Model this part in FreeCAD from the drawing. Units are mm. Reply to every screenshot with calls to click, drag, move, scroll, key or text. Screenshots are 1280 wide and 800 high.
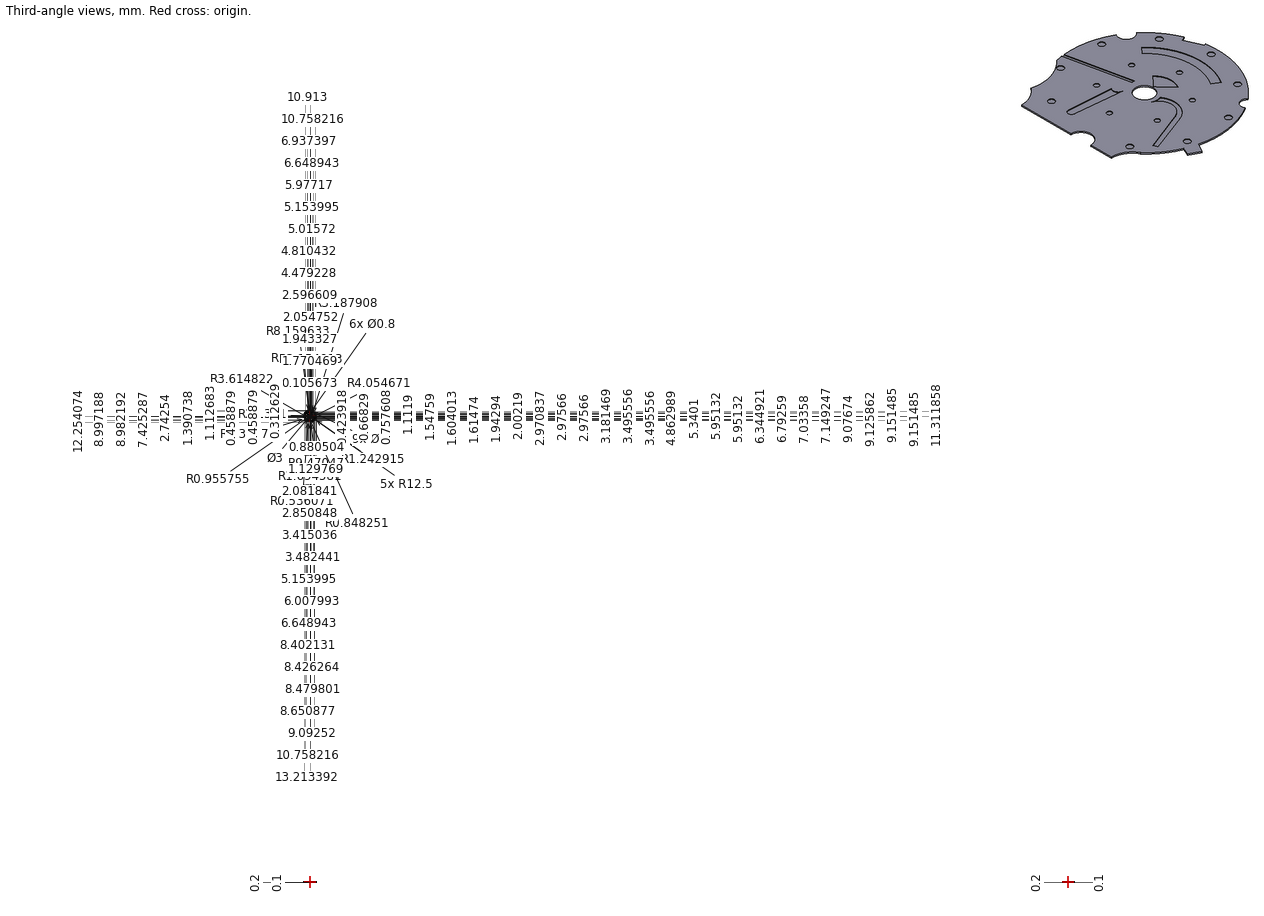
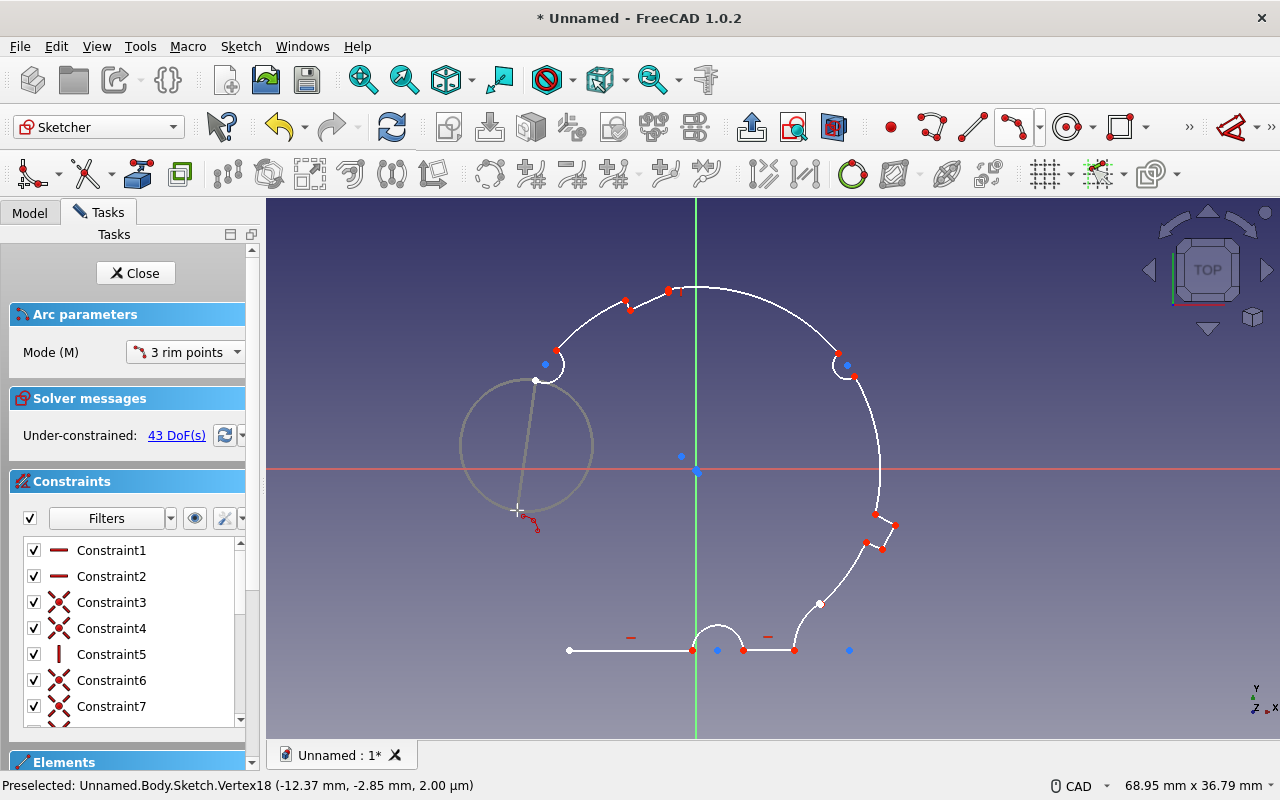
scroll(514, 443, up, 2)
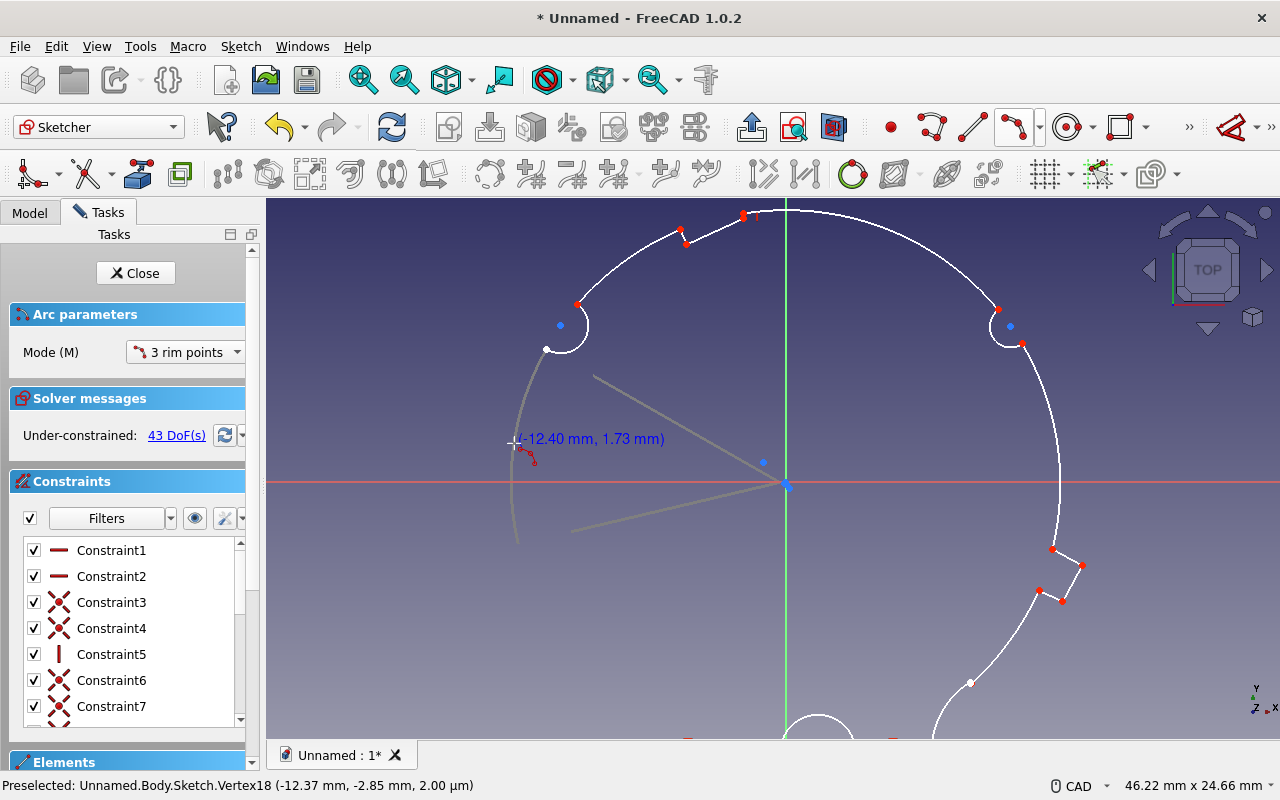
click(515, 443)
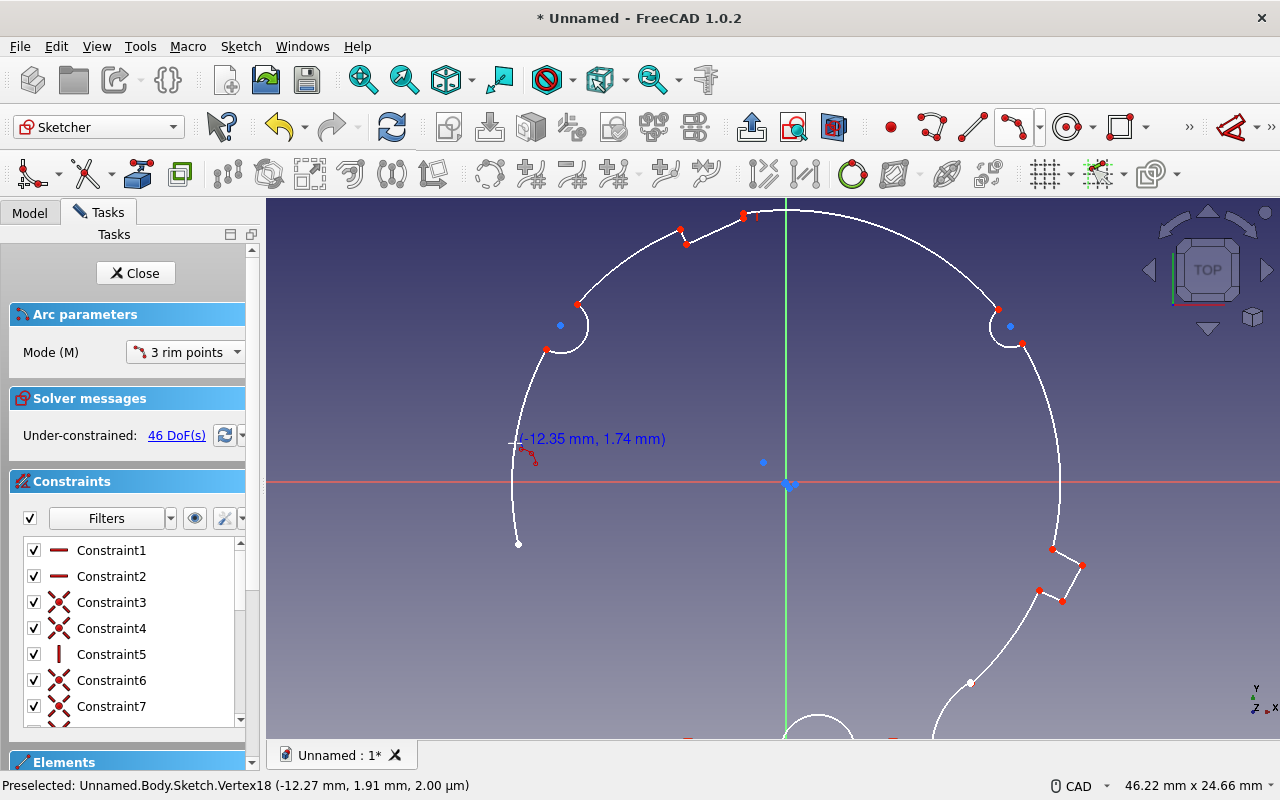
click(518, 544)
click(560, 679)
click(558, 605)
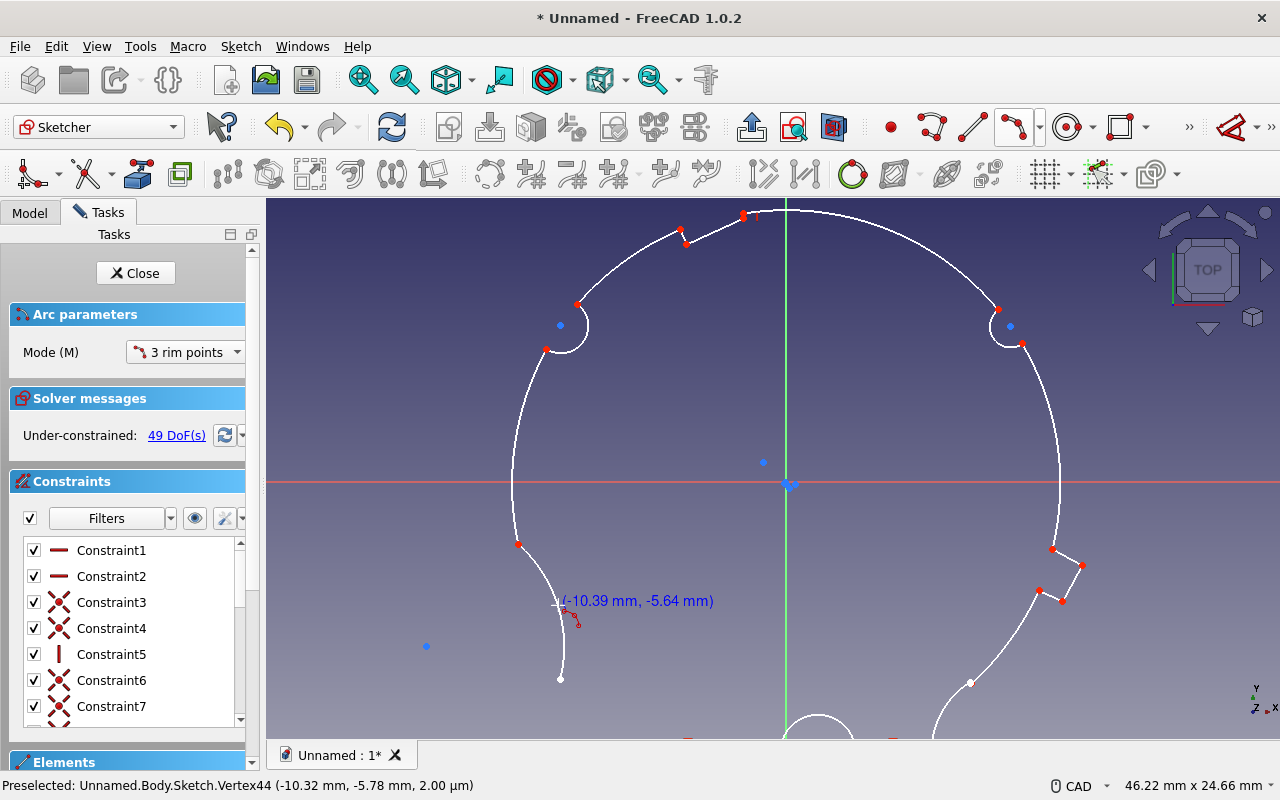
click(560, 680)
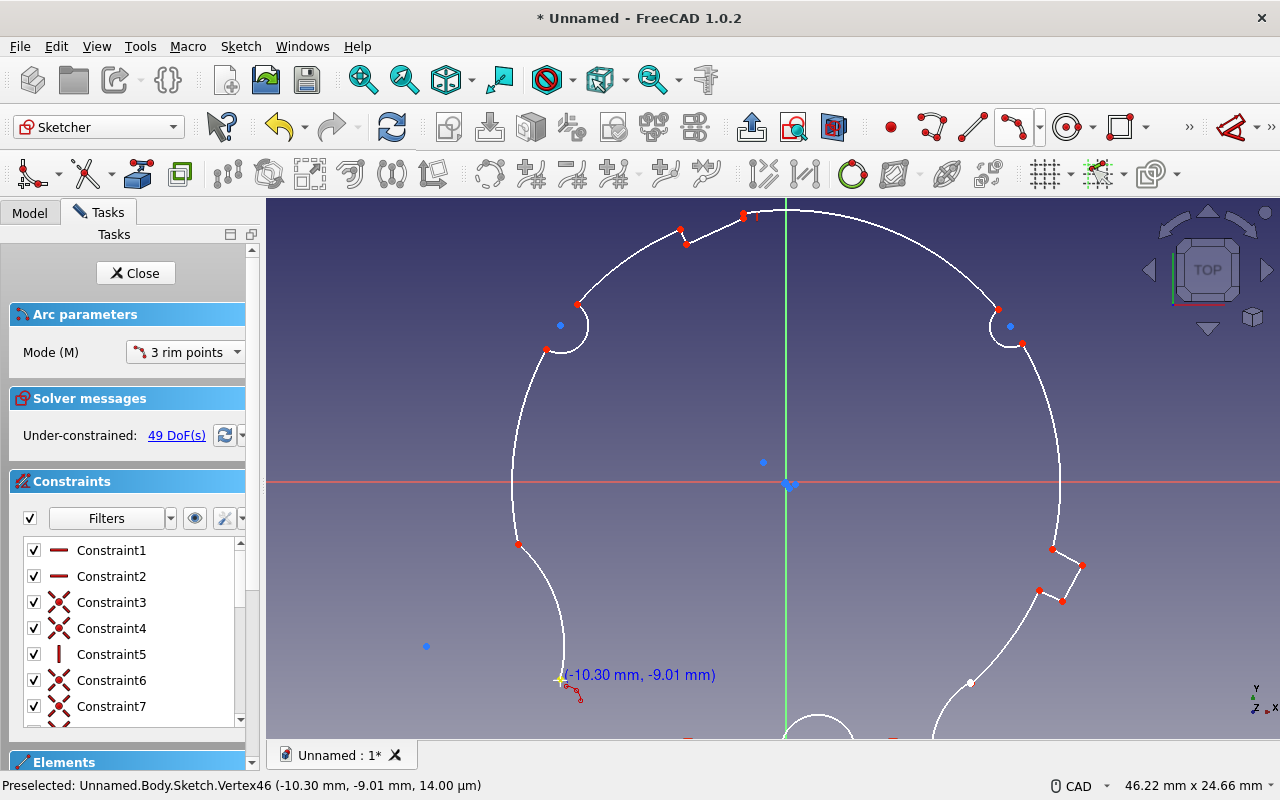
scroll(513, 443, down, 2)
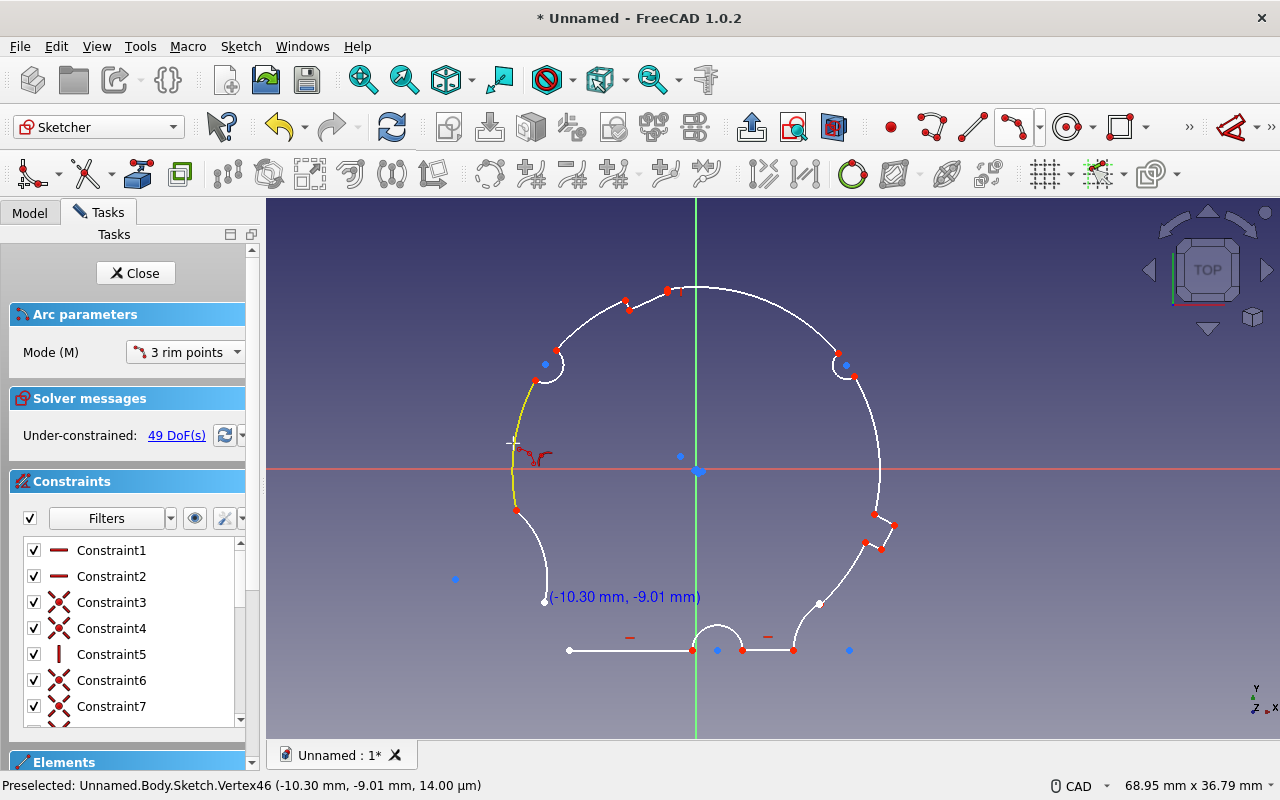
click(569, 651)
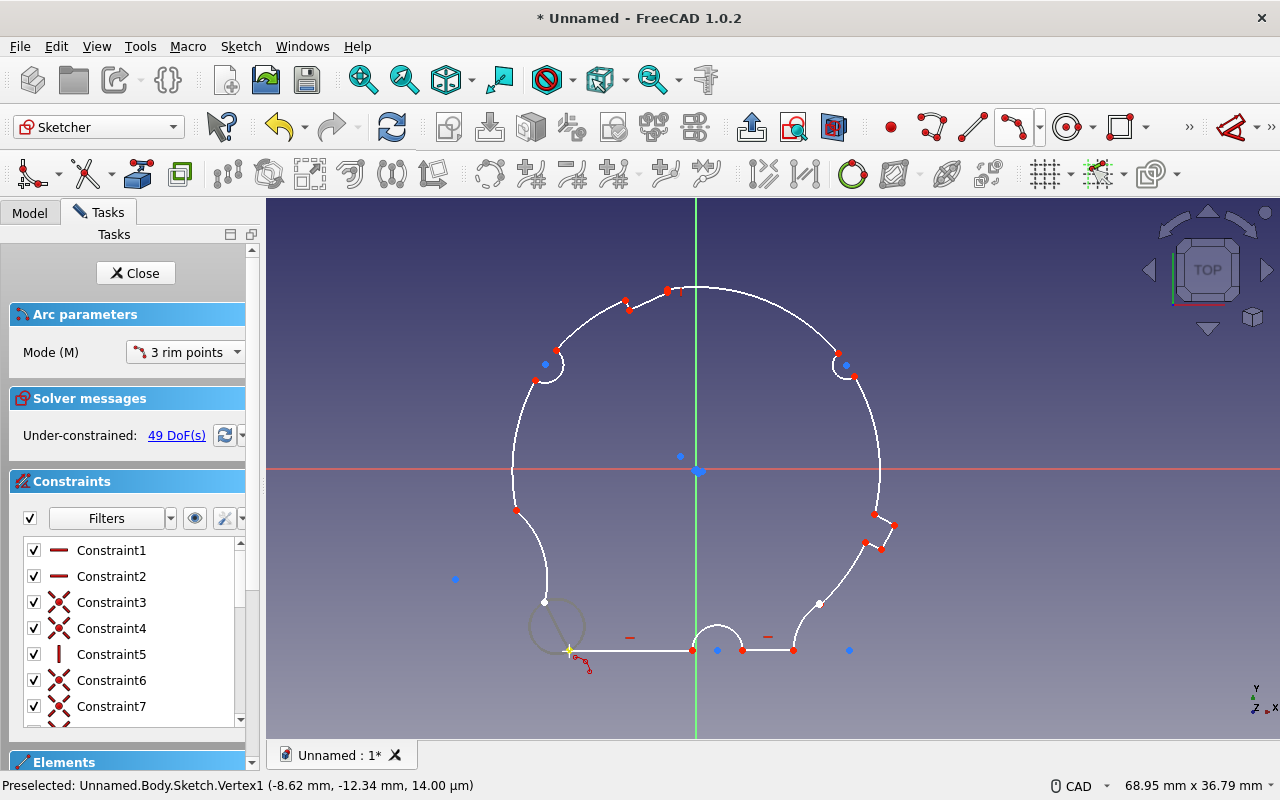
scroll(562, 623, up, 5)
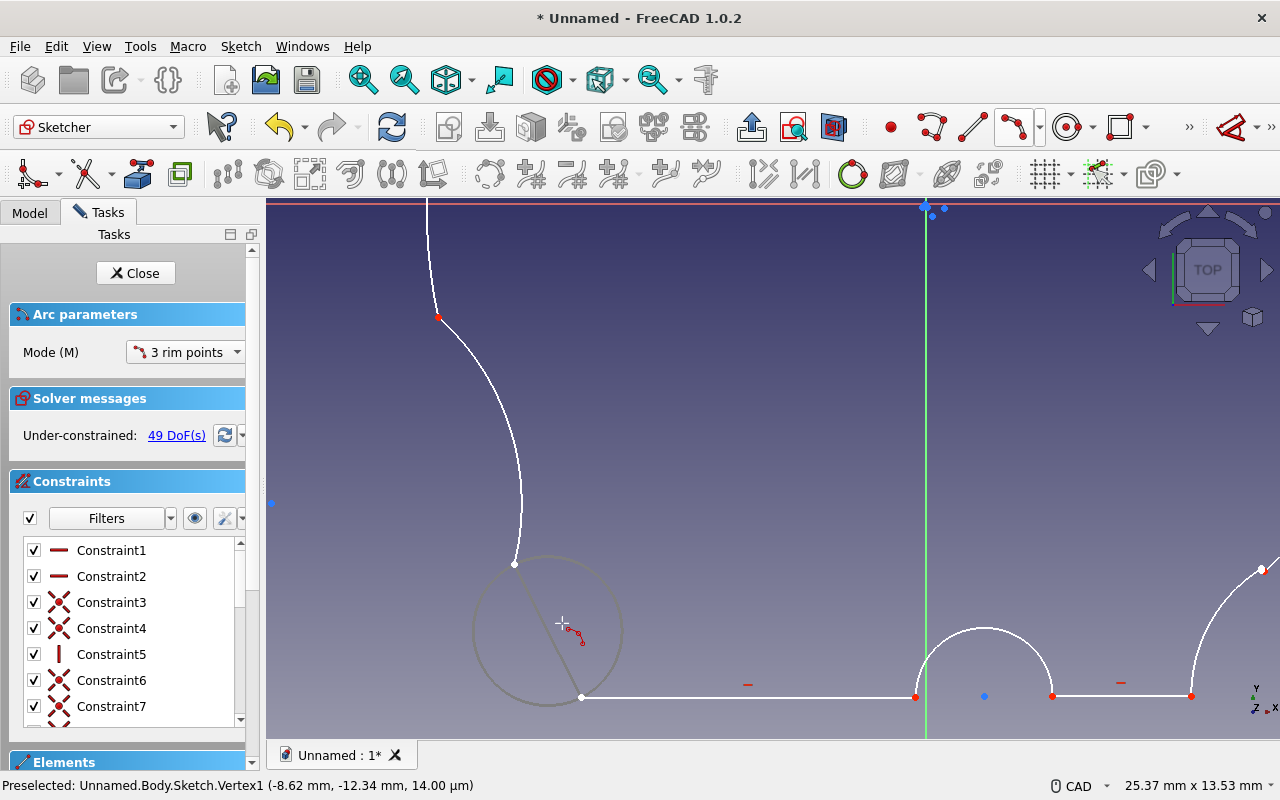
click(562, 621)
key(Escape)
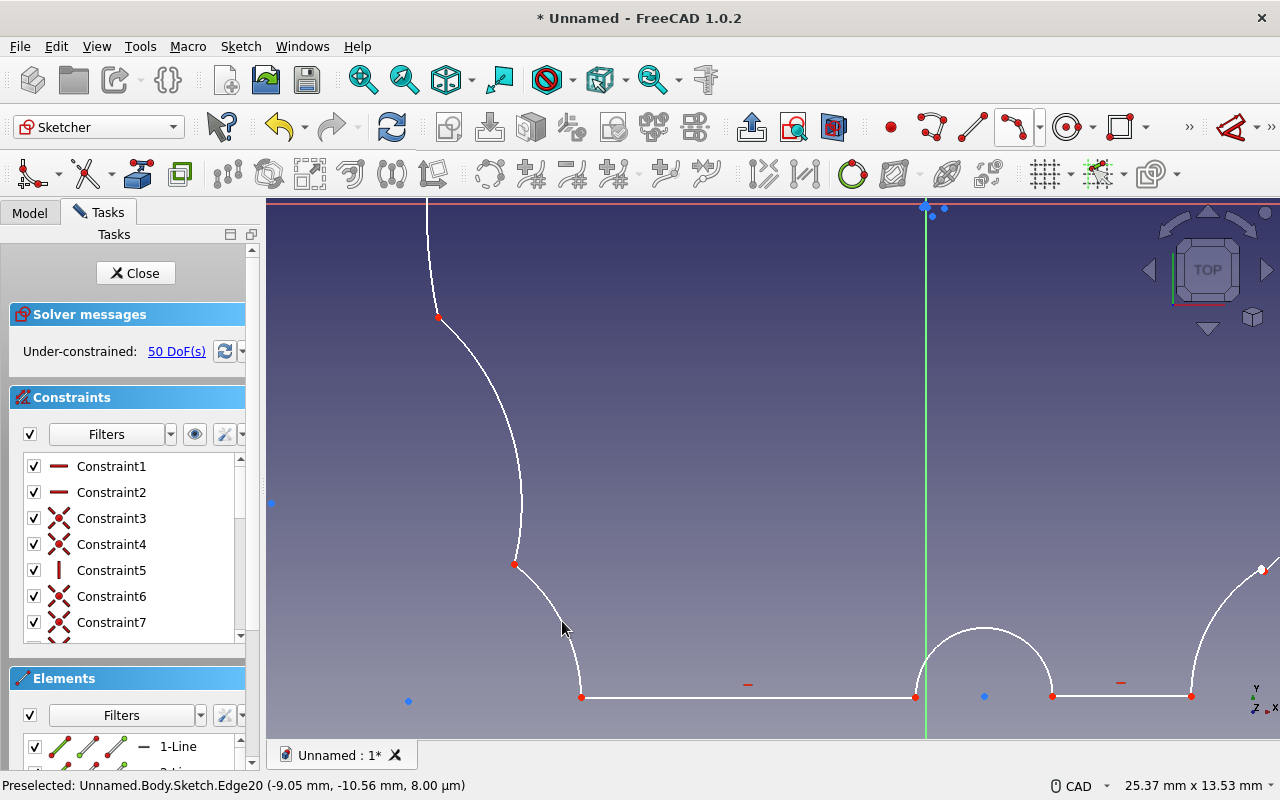
scroll(562, 623, down, 5)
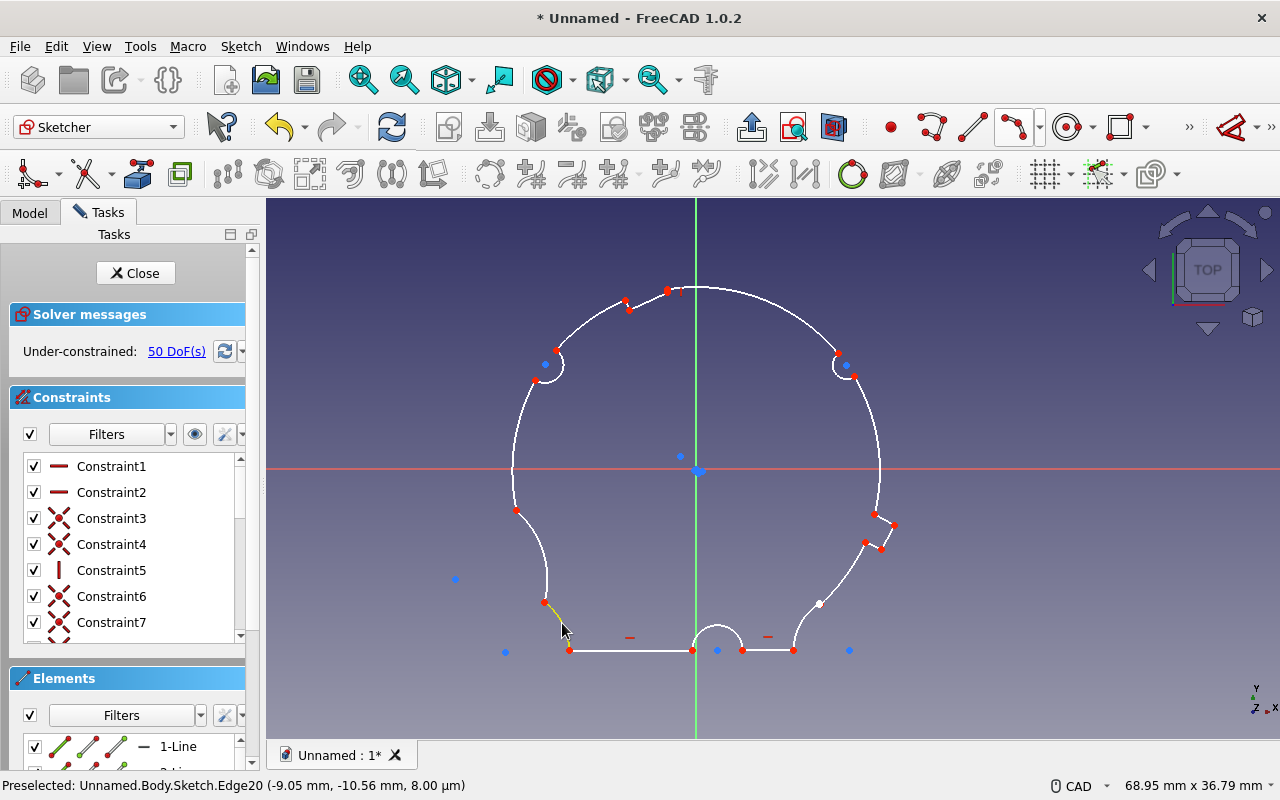
click(837, 588)